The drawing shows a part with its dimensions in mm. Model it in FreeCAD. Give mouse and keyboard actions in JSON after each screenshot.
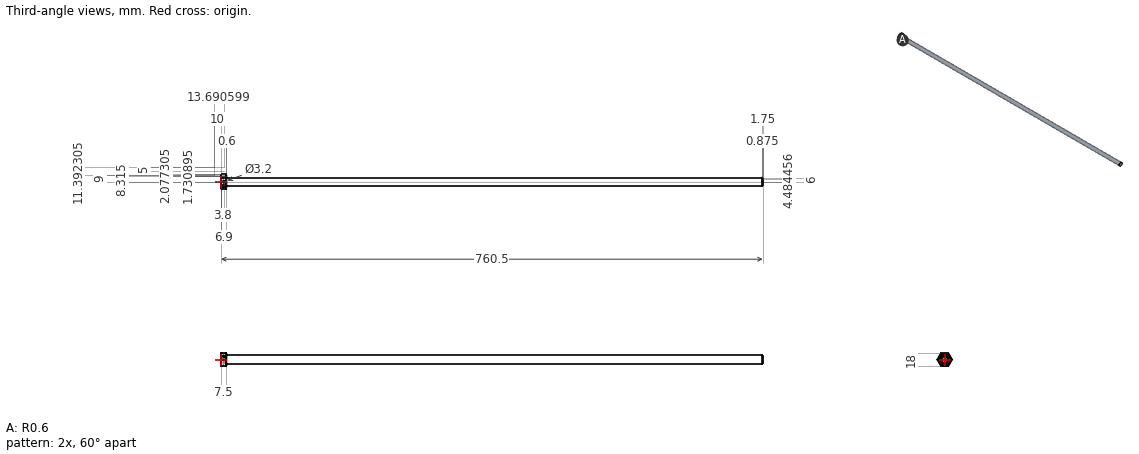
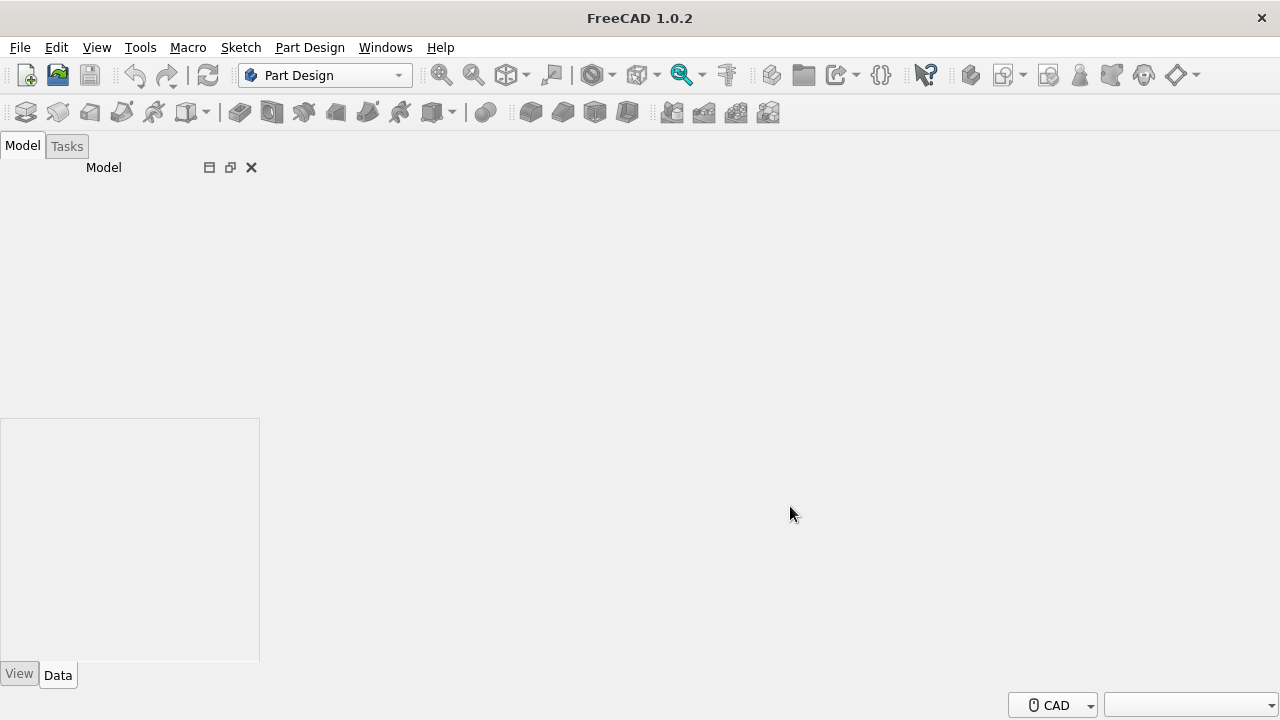
{"action": "key", "text": "ctrl+n"}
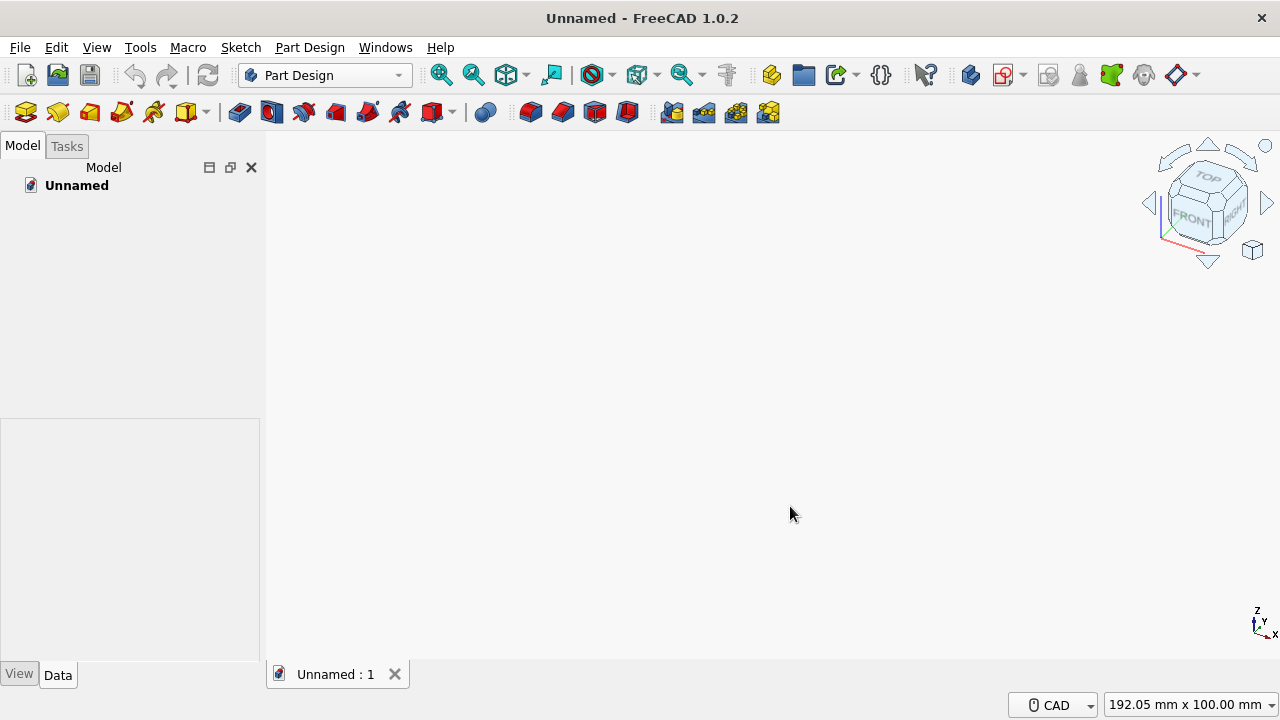
{"action": "left_click", "coordinate": [1004, 76]}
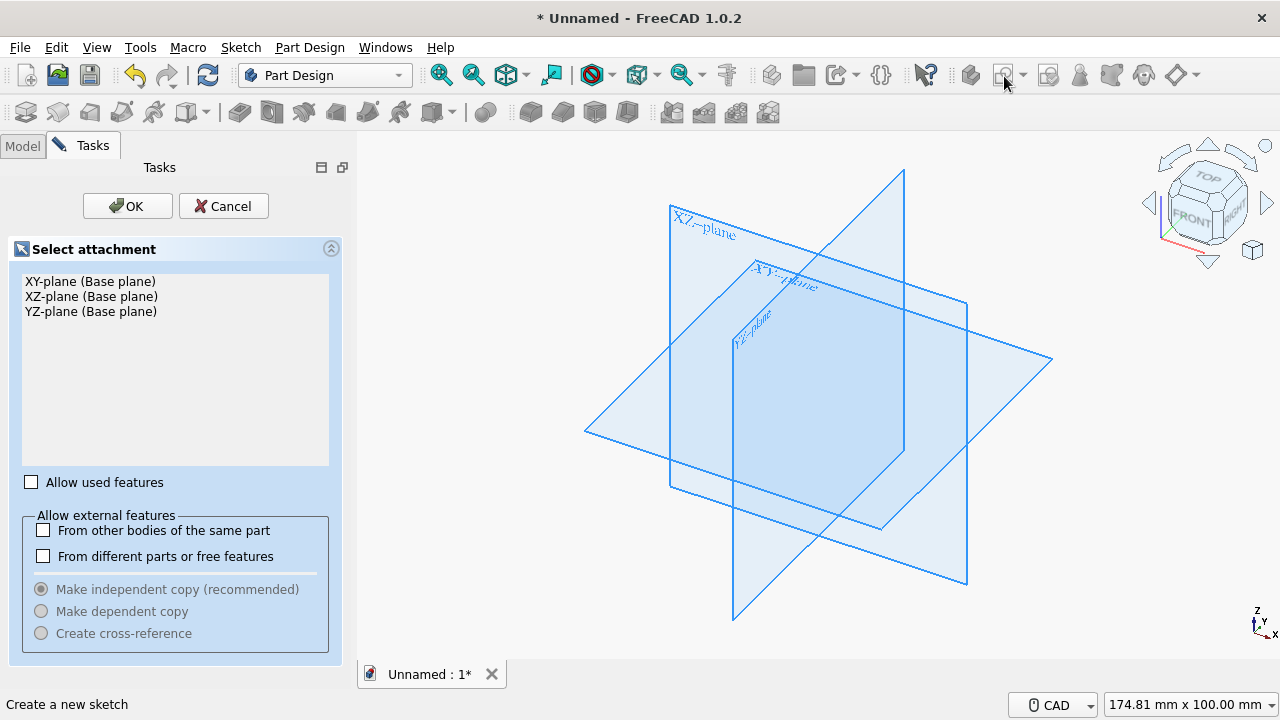
{"action": "left_click", "coordinate": [82, 312]}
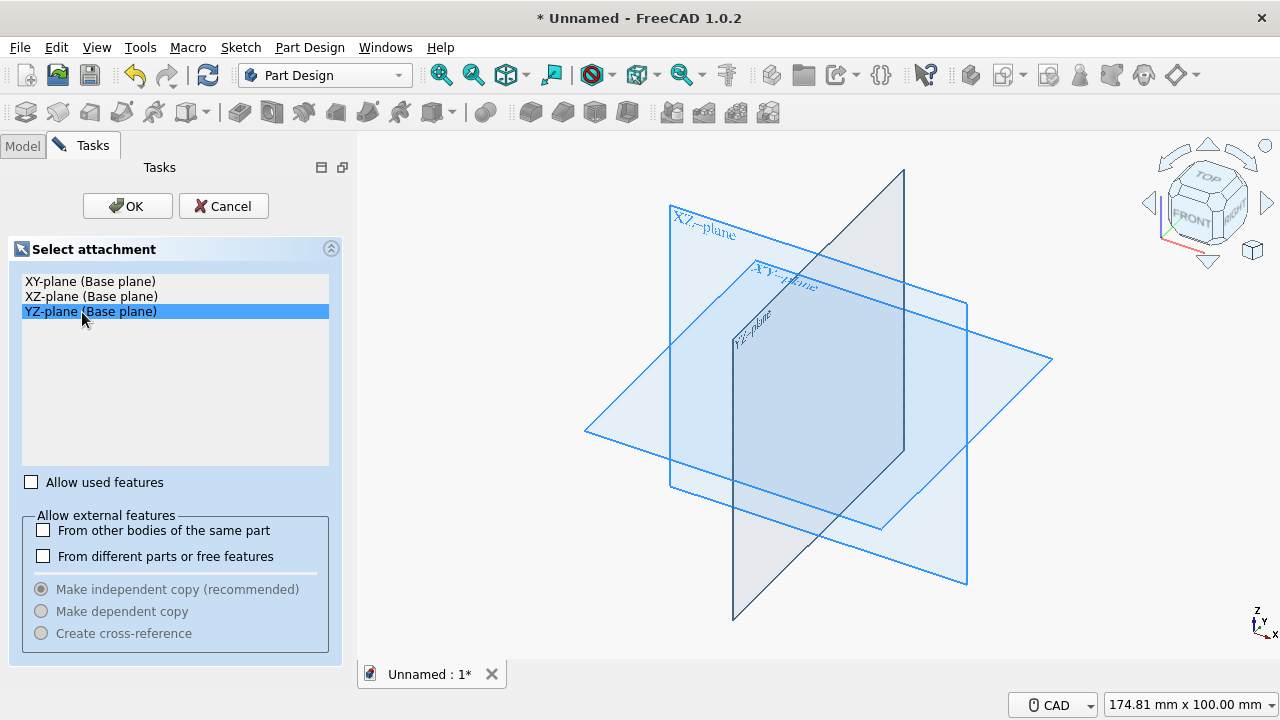
{"action": "left_click", "coordinate": [128, 206]}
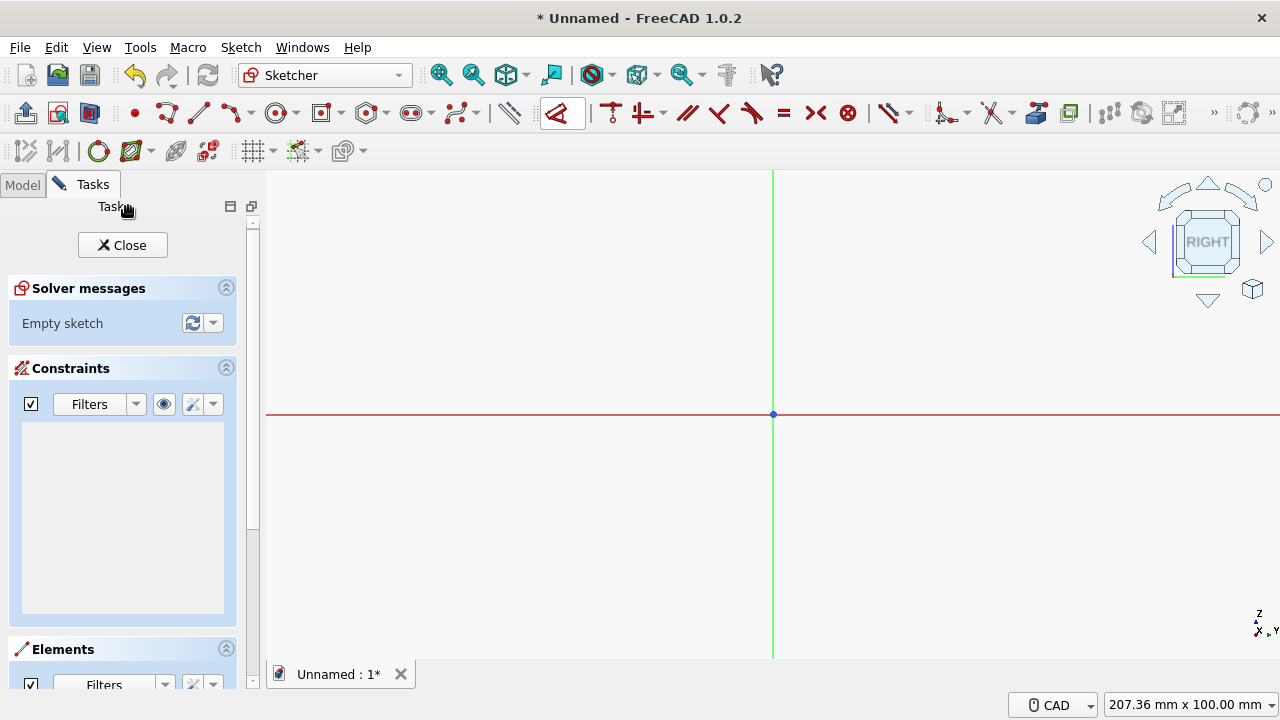
{"action": "scroll", "coordinate": [803, 415], "scroll_direction": "up", "scroll_amount": 6}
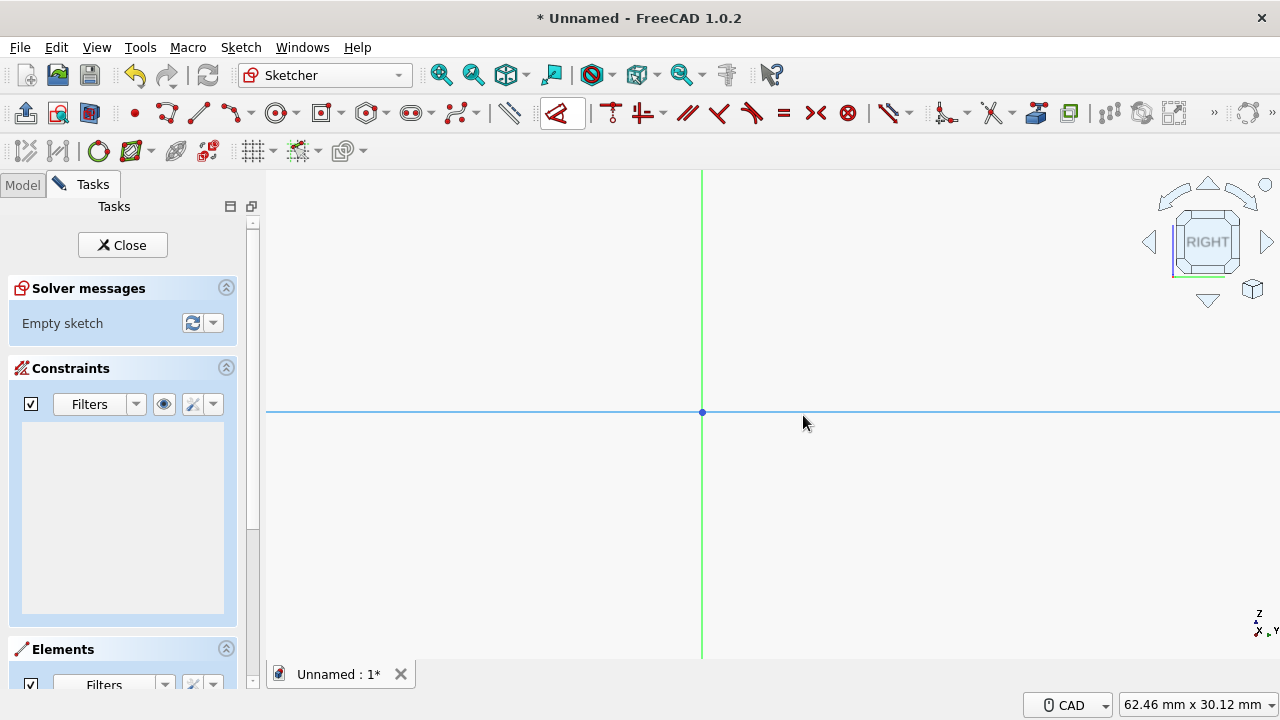
{"action": "key", "text": "g p 6"}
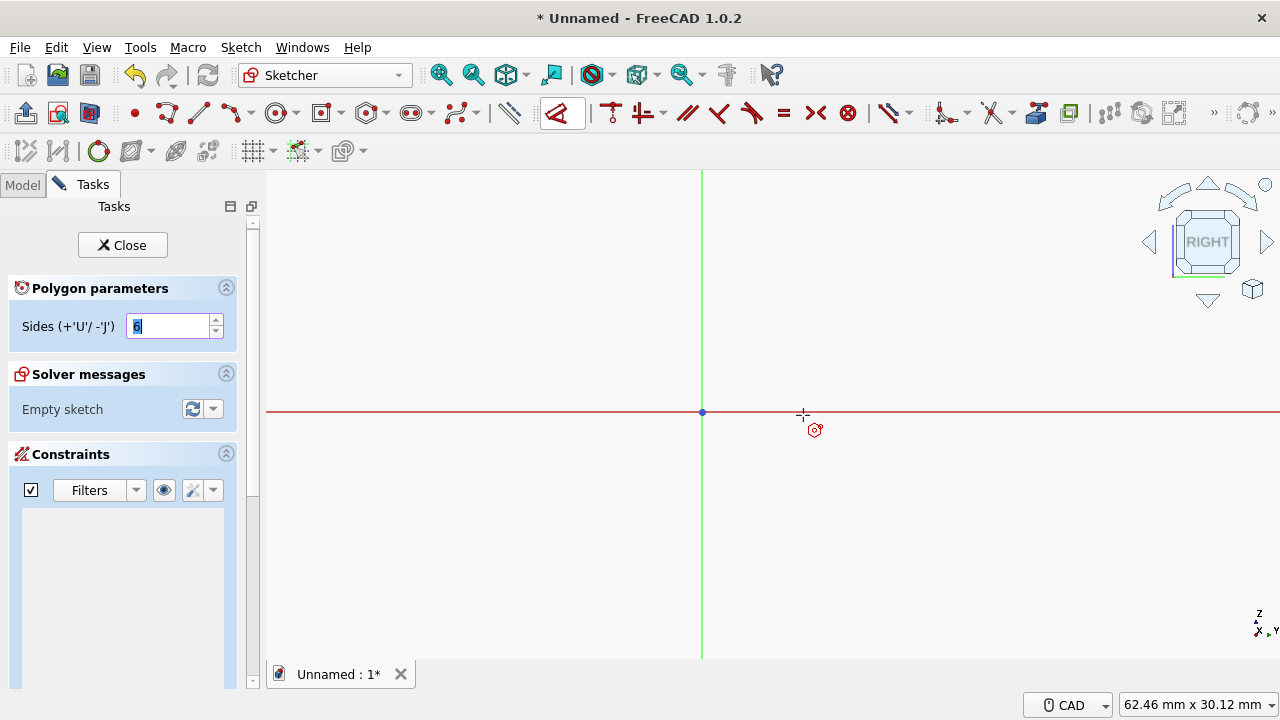
{"action": "left_click", "coordinate": [702, 412]}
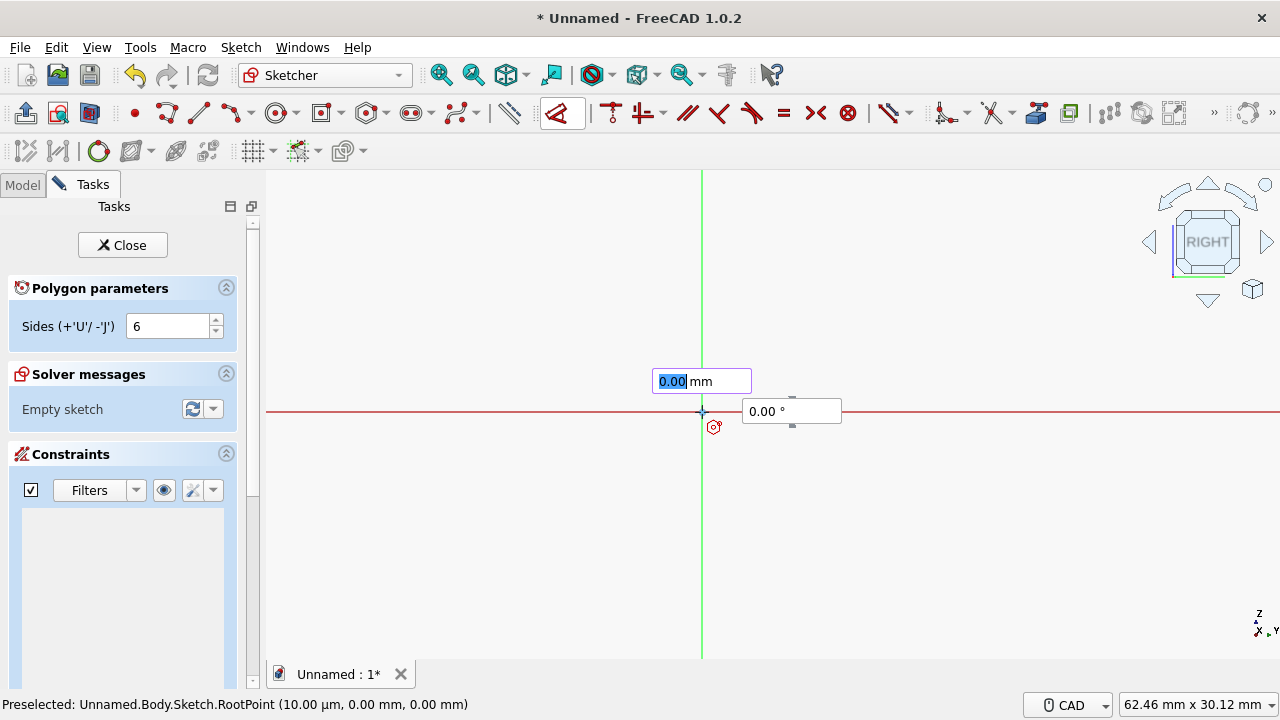
{"action": "left_click", "coordinate": [871, 412]}
{"action": "right_click", "coordinate": [871, 412]}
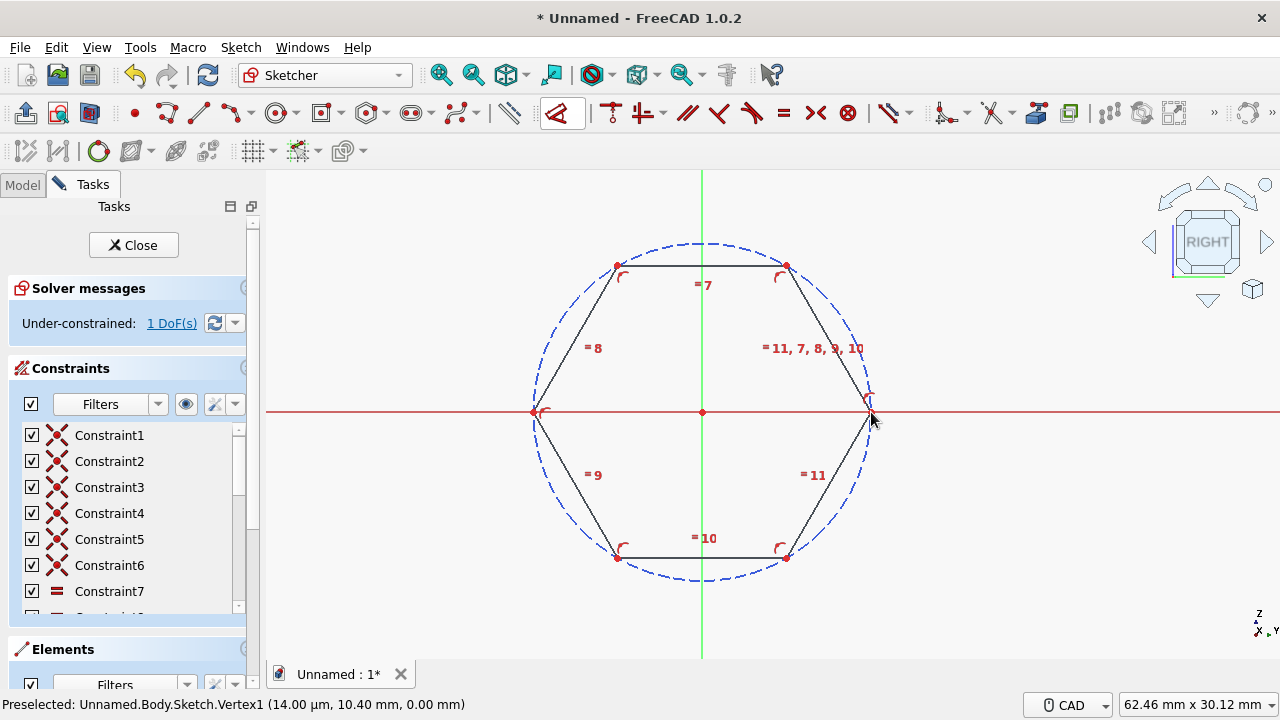
{"action": "left_click", "coordinate": [556, 114]}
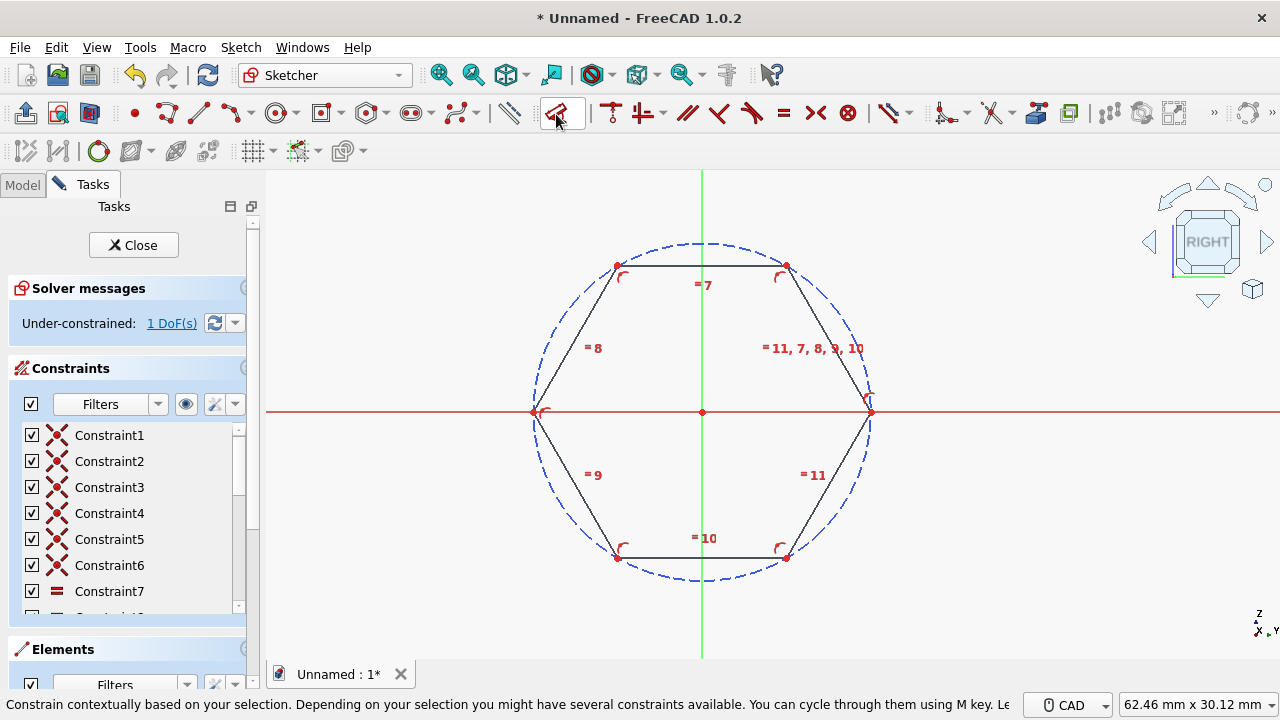
{"action": "left_click", "coordinate": [618, 558]}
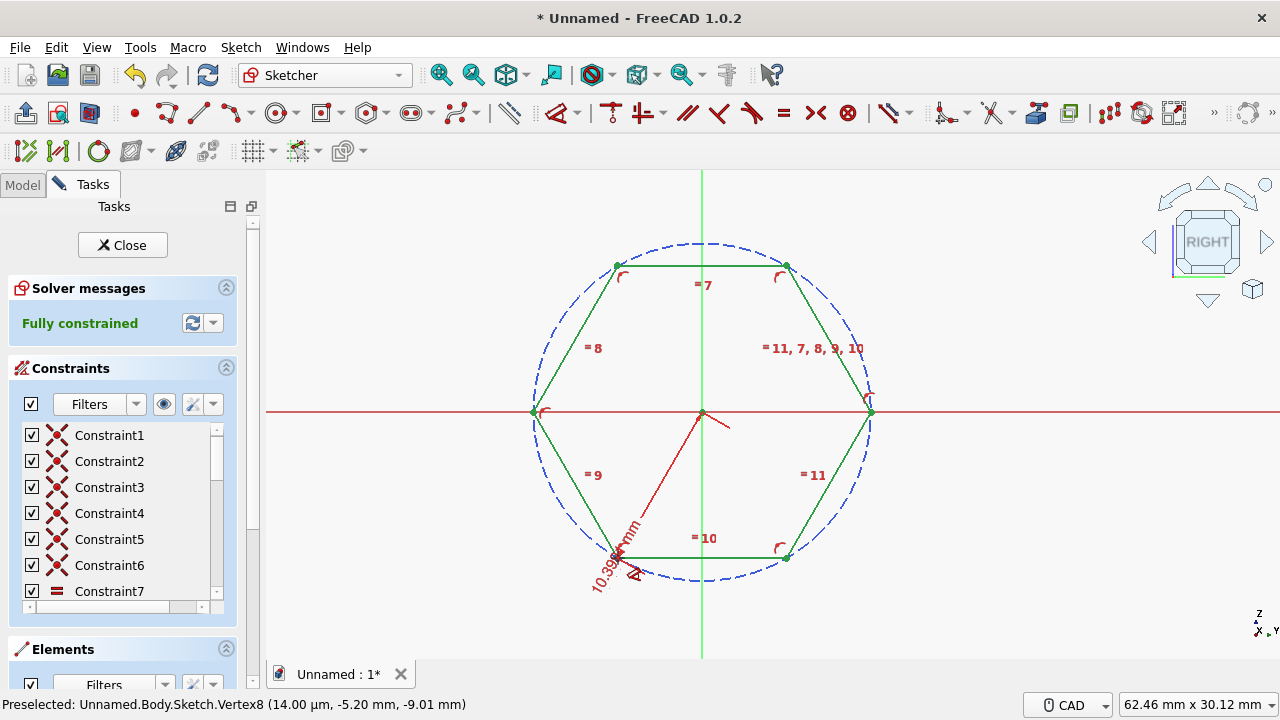
{"action": "left_click", "coordinate": [787, 266]}
{"action": "left_click", "coordinate": [869, 310]}